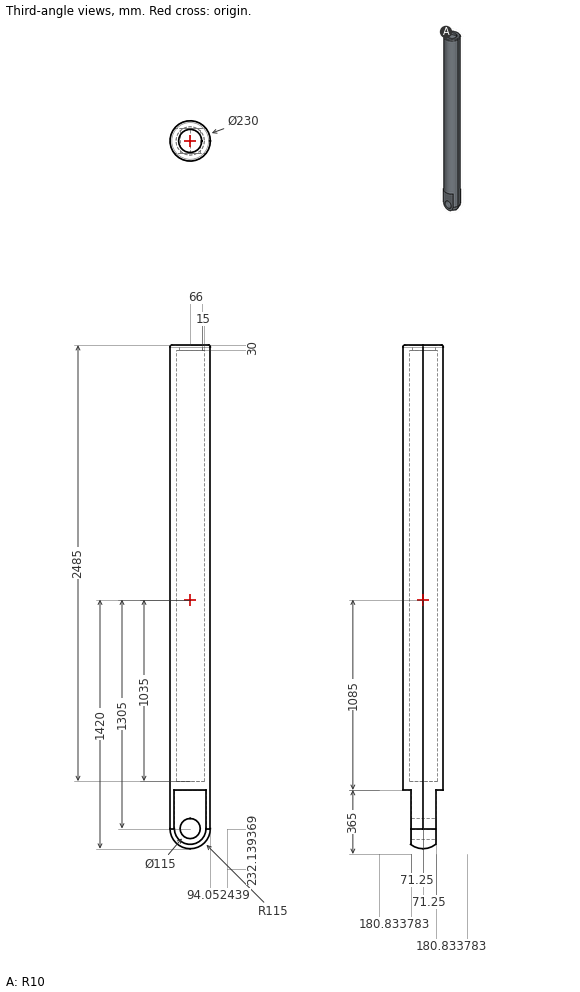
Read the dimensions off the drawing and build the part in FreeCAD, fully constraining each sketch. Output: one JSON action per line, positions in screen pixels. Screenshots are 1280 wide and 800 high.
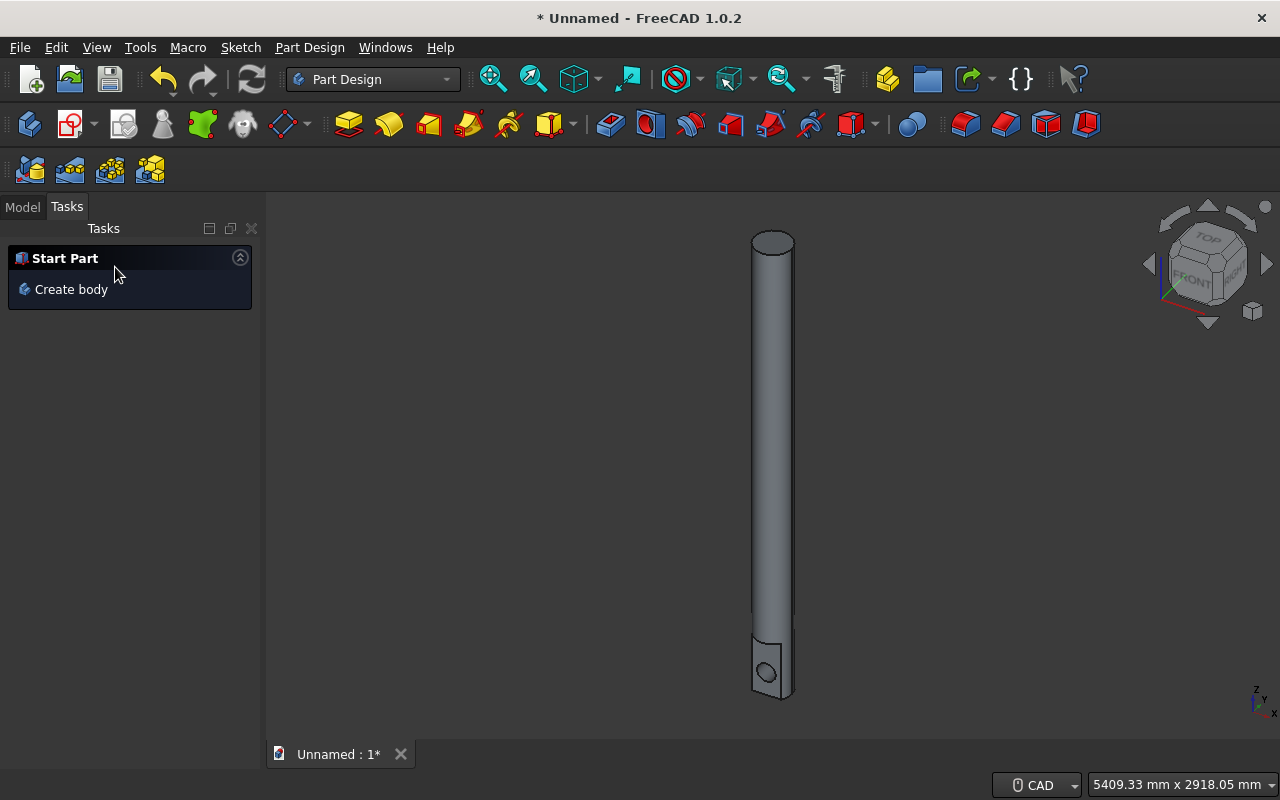
{"action": "left_click", "coordinate": [70, 124]}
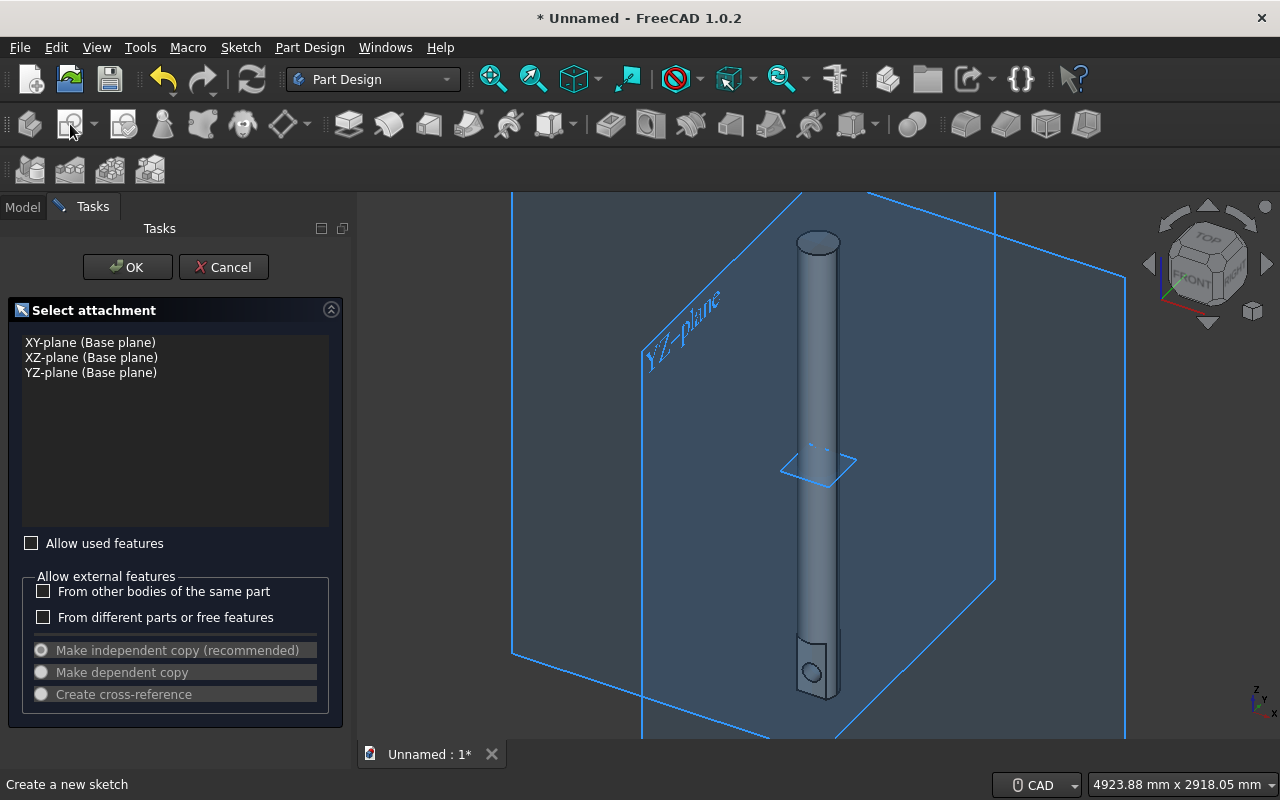
{"action": "left_click", "coordinate": [82, 358]}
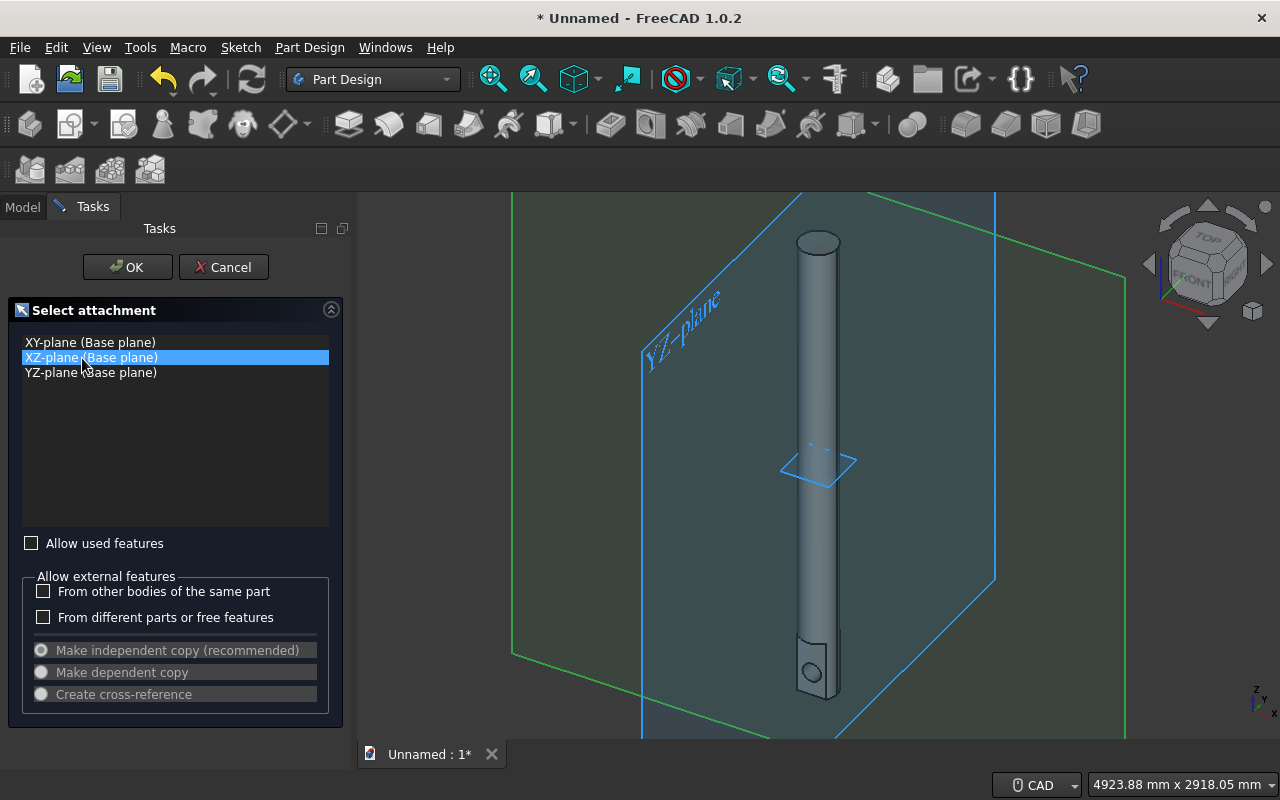
{"action": "left_click", "coordinate": [128, 267]}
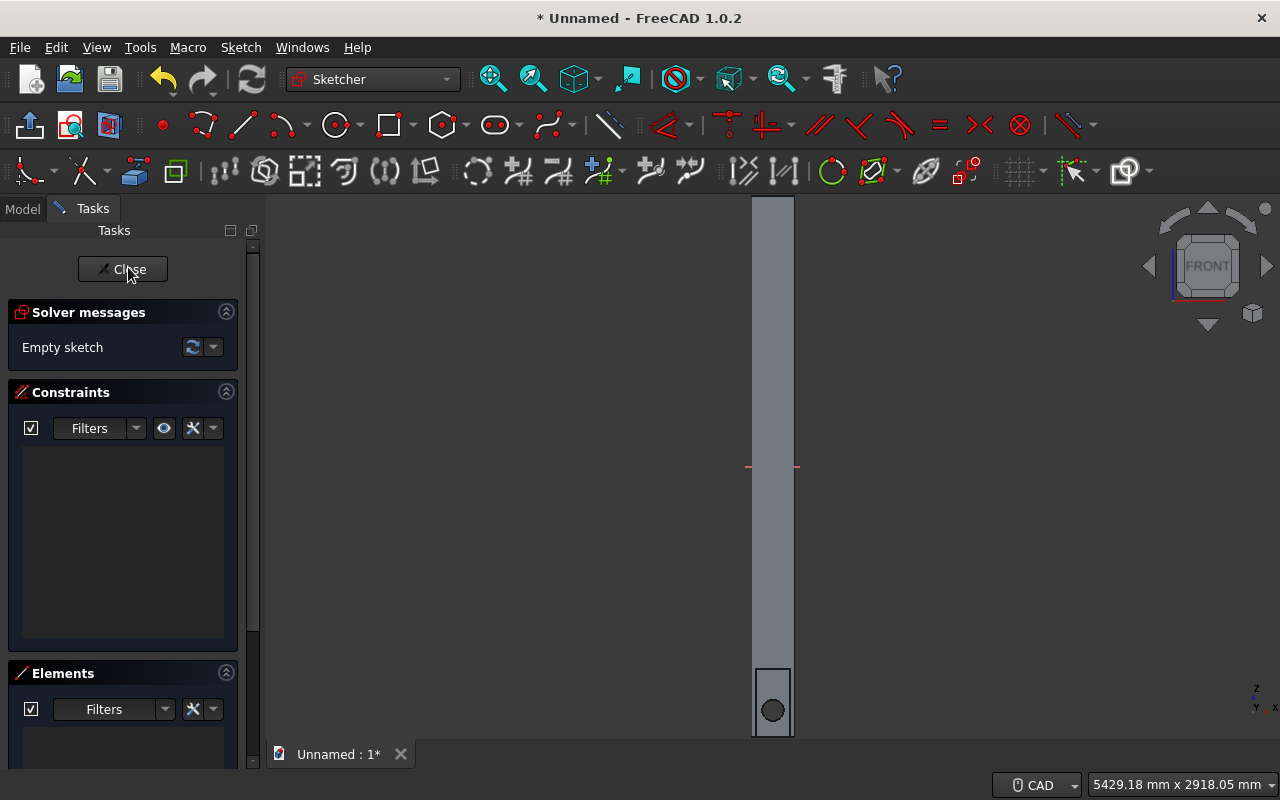
{"action": "key", "text": "q s"}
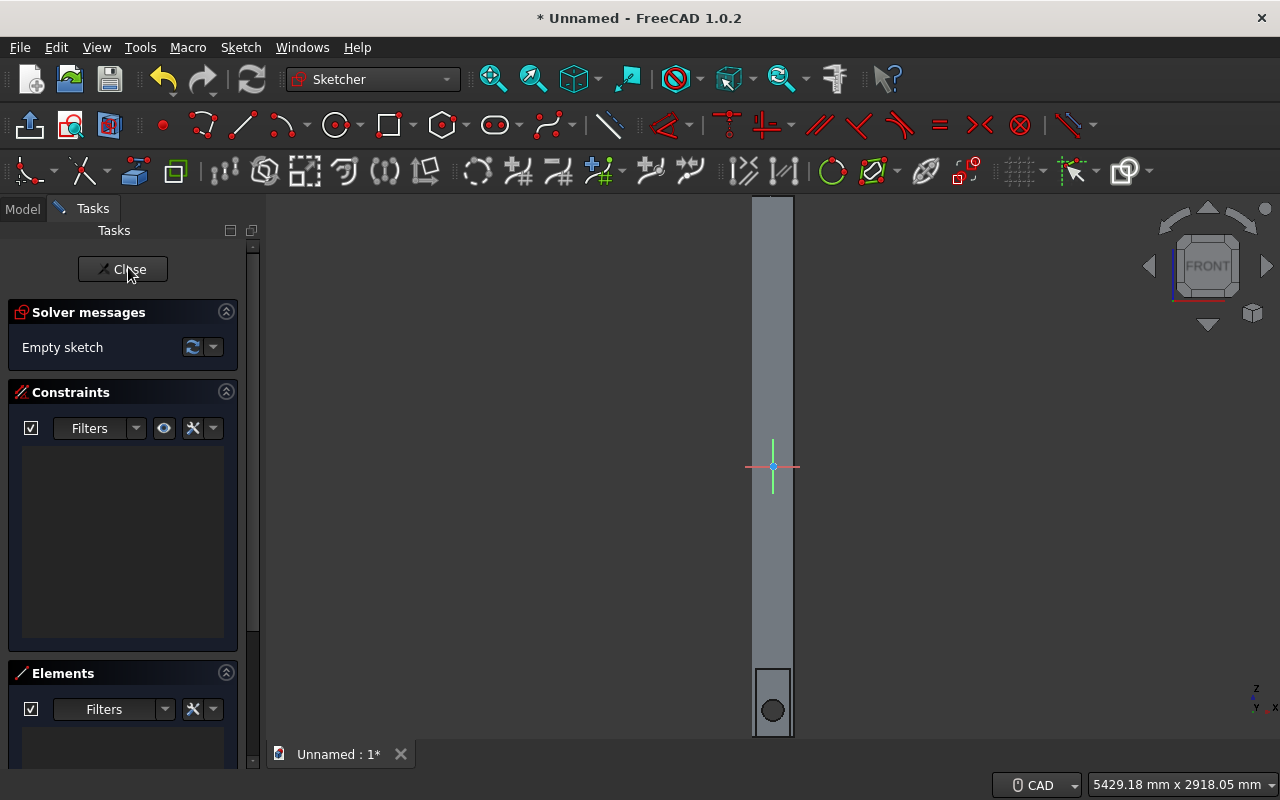
{"action": "scroll", "coordinate": [704, 466], "scroll_direction": "down", "scroll_amount": 5}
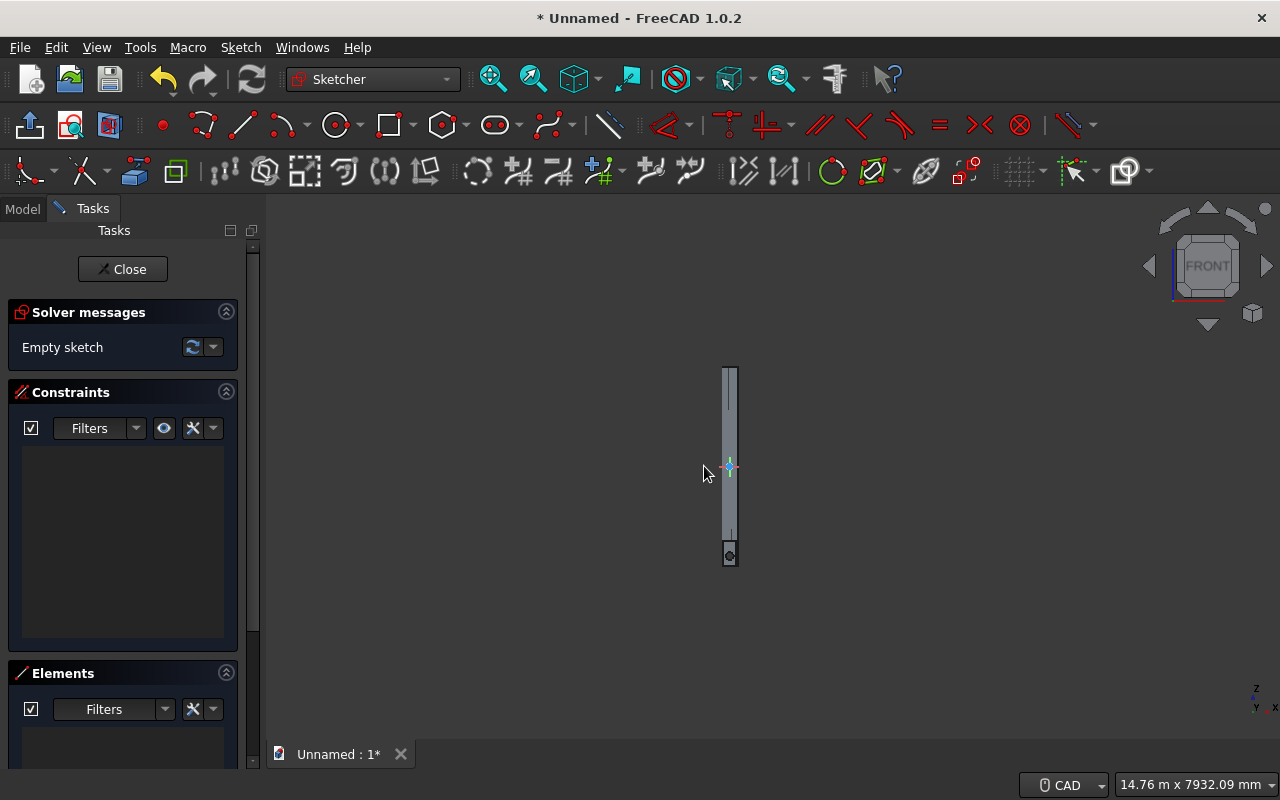
{"action": "scroll", "coordinate": [739, 569], "scroll_direction": "up", "scroll_amount": 15}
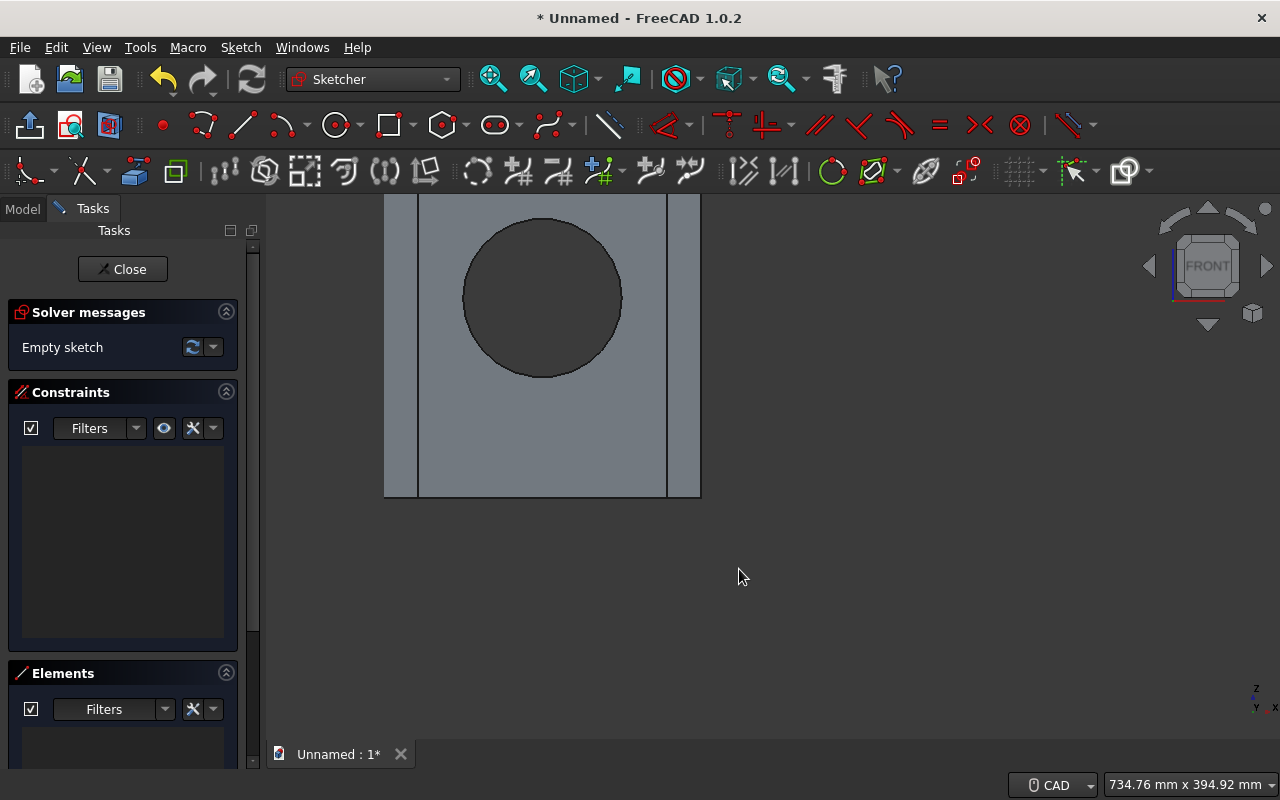
{"action": "key", "text": "g m"}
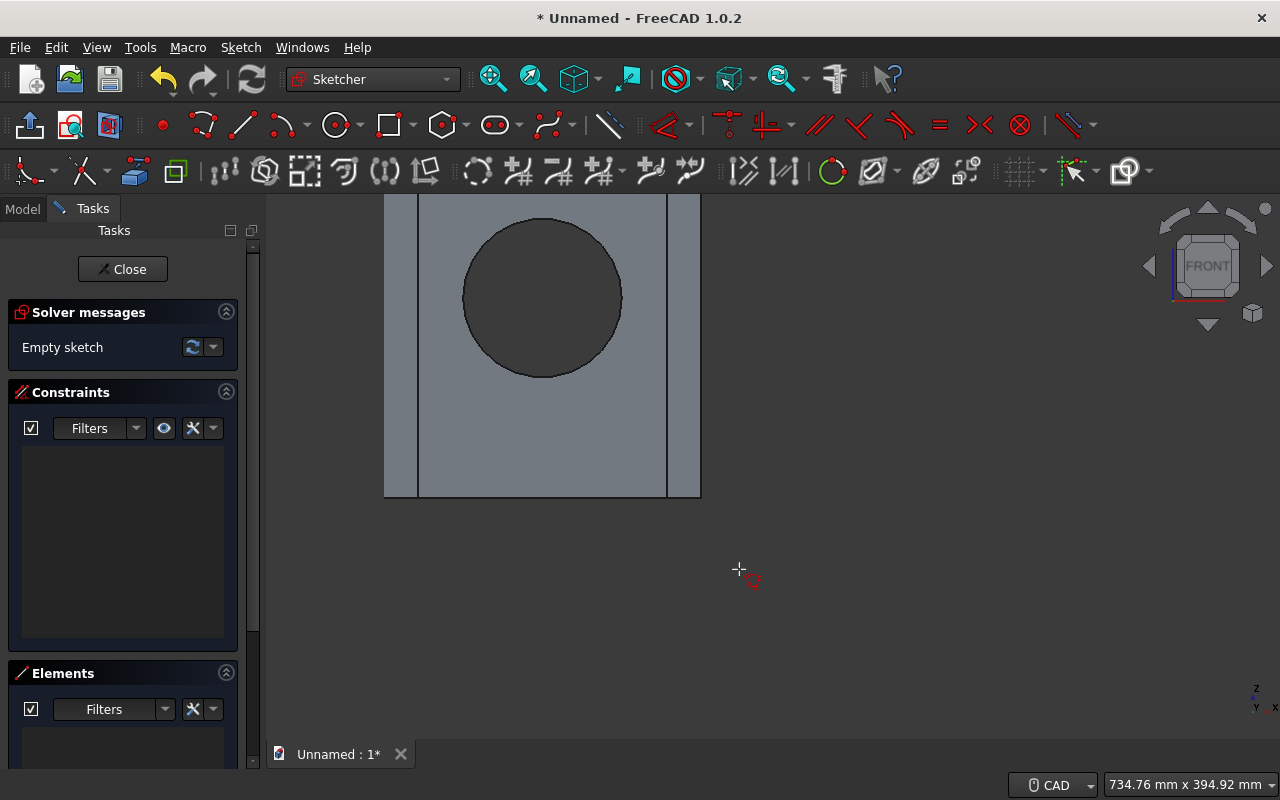
{"action": "left_click", "coordinate": [701, 298]}
{"action": "left_click", "coordinate": [831, 298]}
{"action": "left_click", "coordinate": [831, 618]}
{"action": "left_click", "coordinate": [542, 618]}
{"action": "left_click", "coordinate": [551, 457]}
{"action": "right_click", "coordinate": [551, 457]}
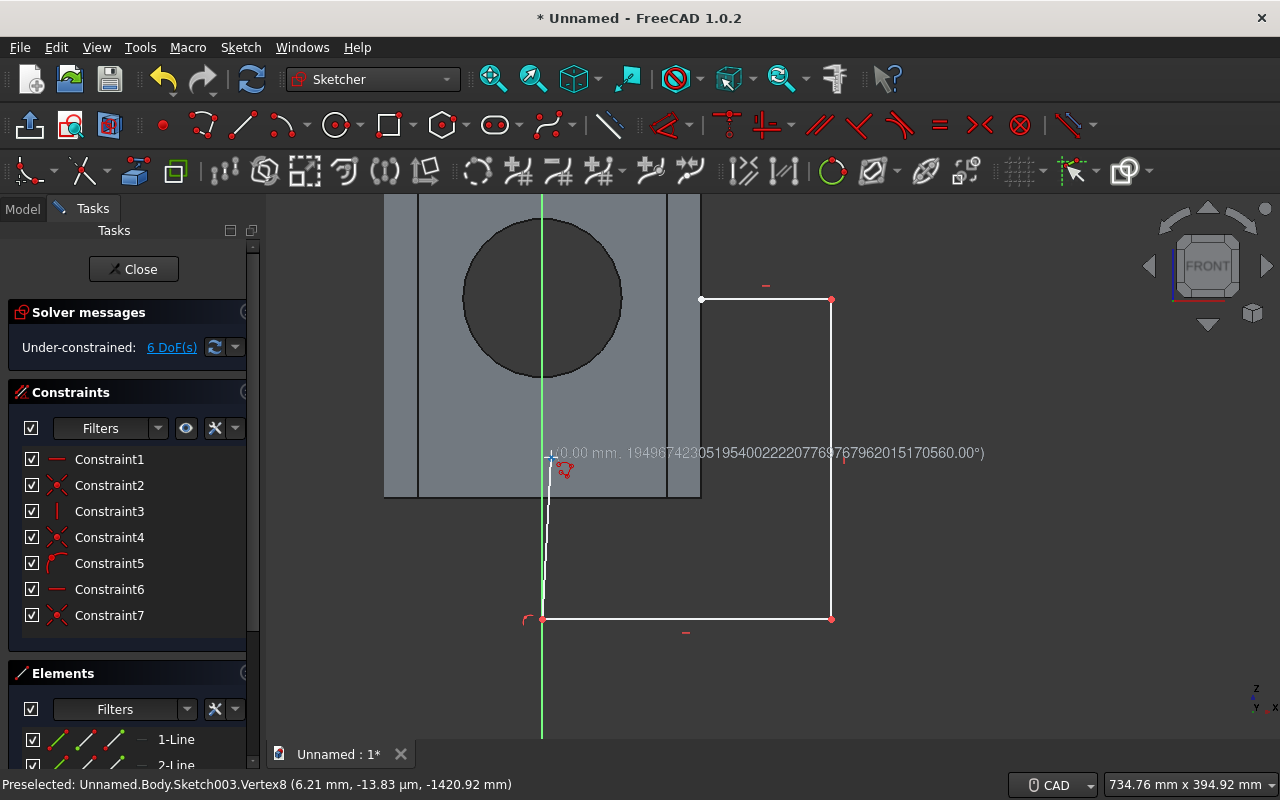
{"action": "left_click", "coordinate": [310, 126]}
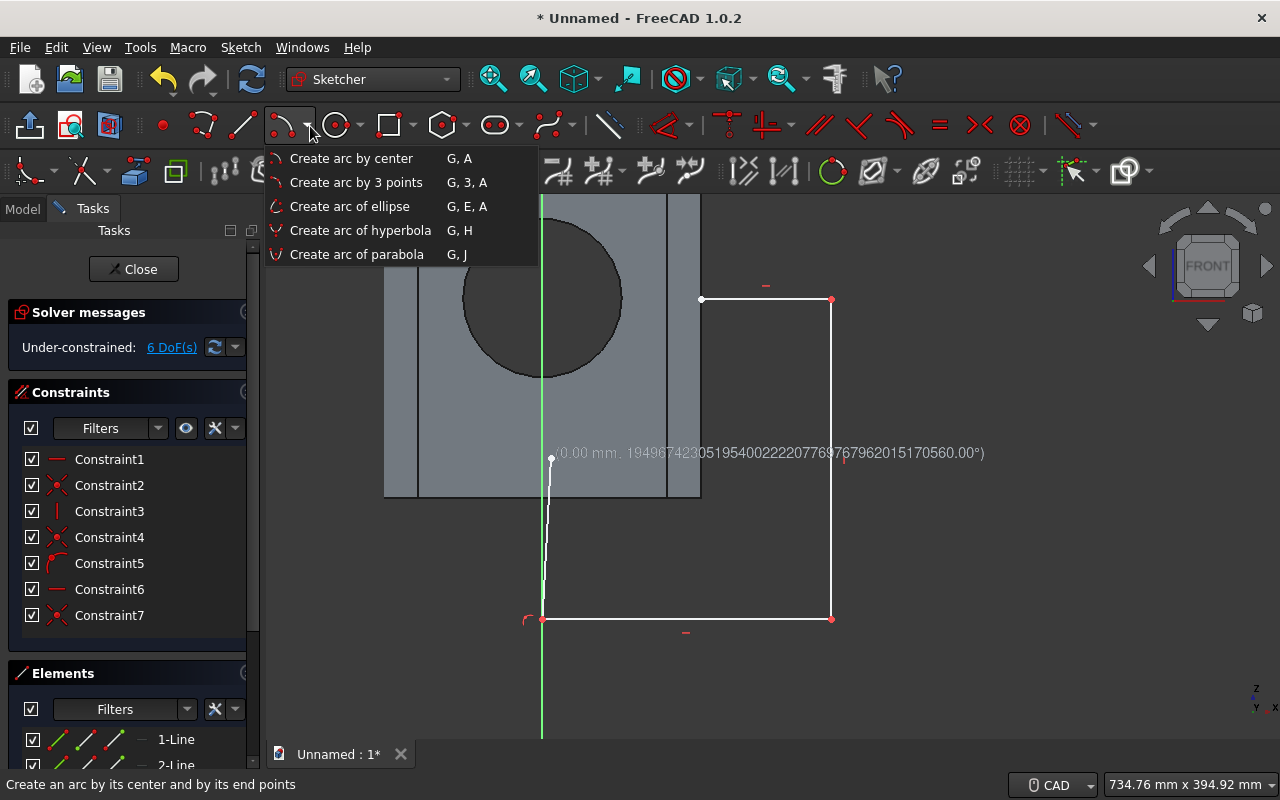
{"action": "left_click", "coordinate": [402, 182]}